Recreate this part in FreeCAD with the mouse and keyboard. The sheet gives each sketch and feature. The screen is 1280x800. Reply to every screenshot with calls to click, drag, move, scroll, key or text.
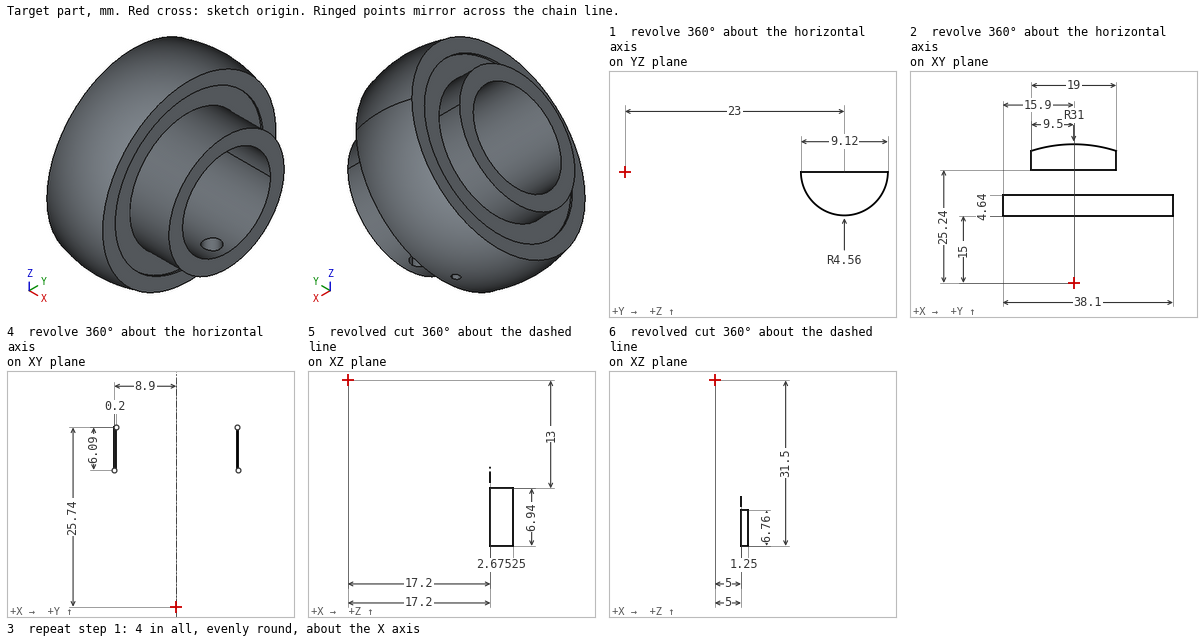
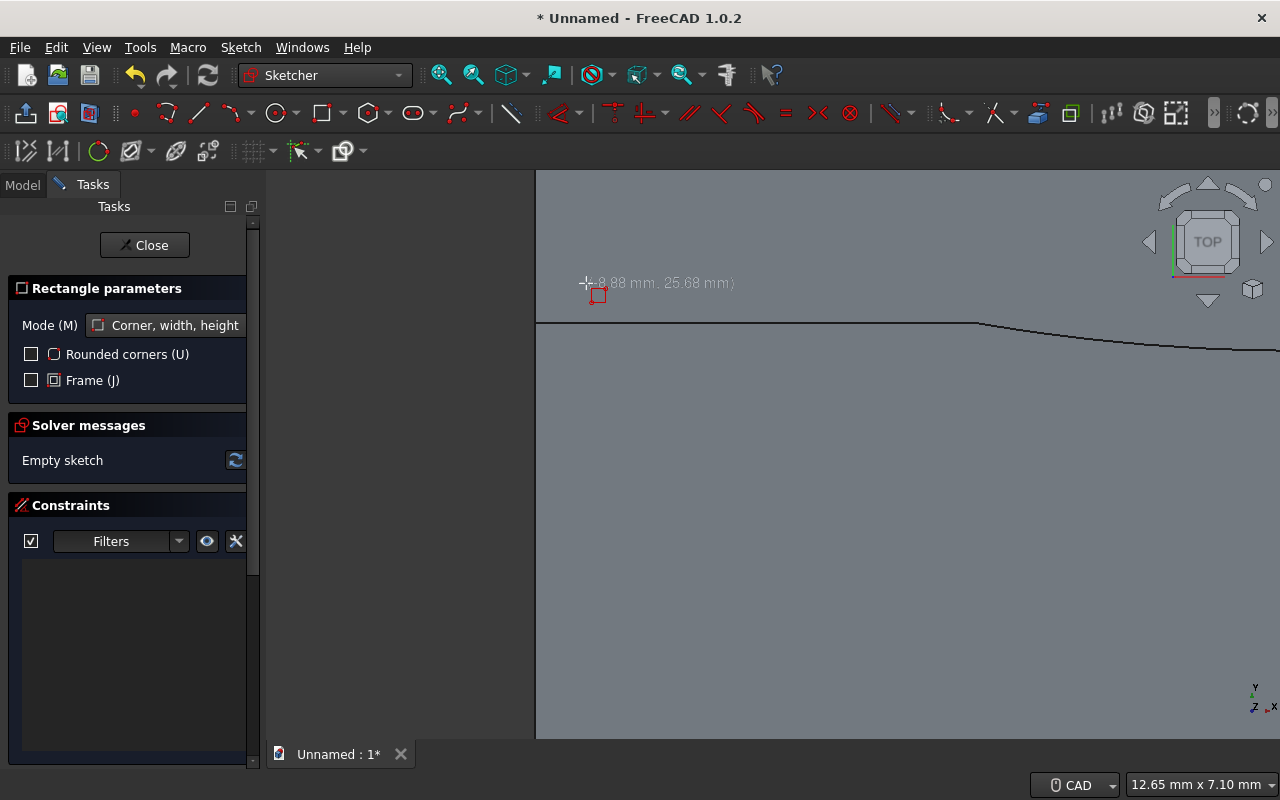
scroll(587, 284, down, 9)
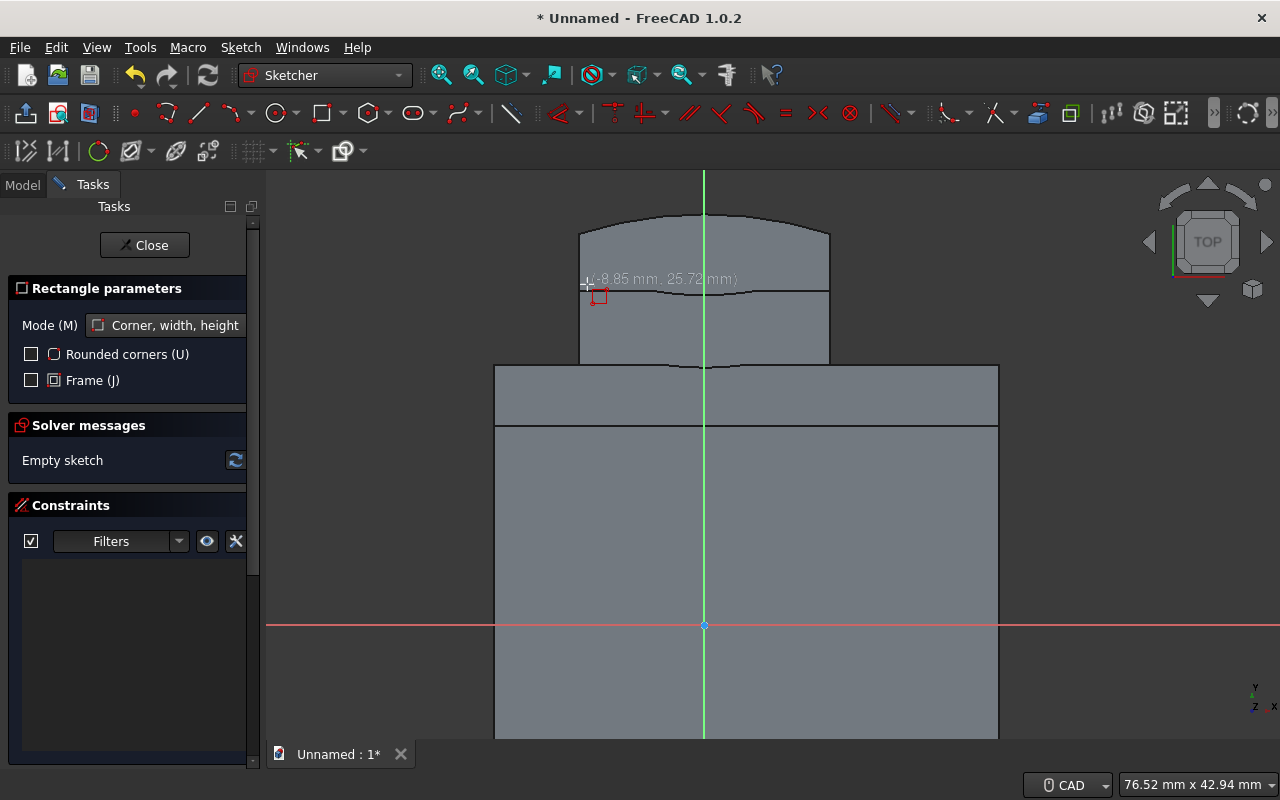
click(587, 284)
click(589, 365)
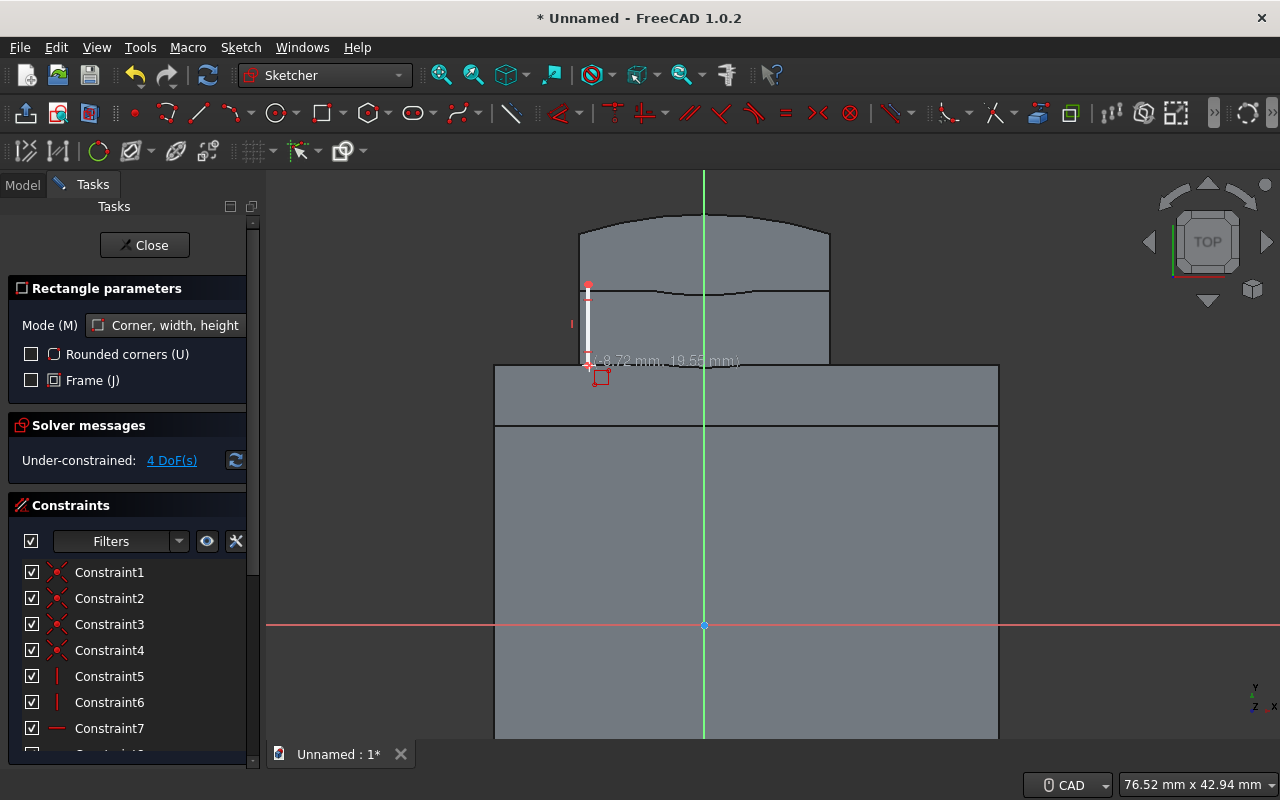
scroll(820, 284, up, 9)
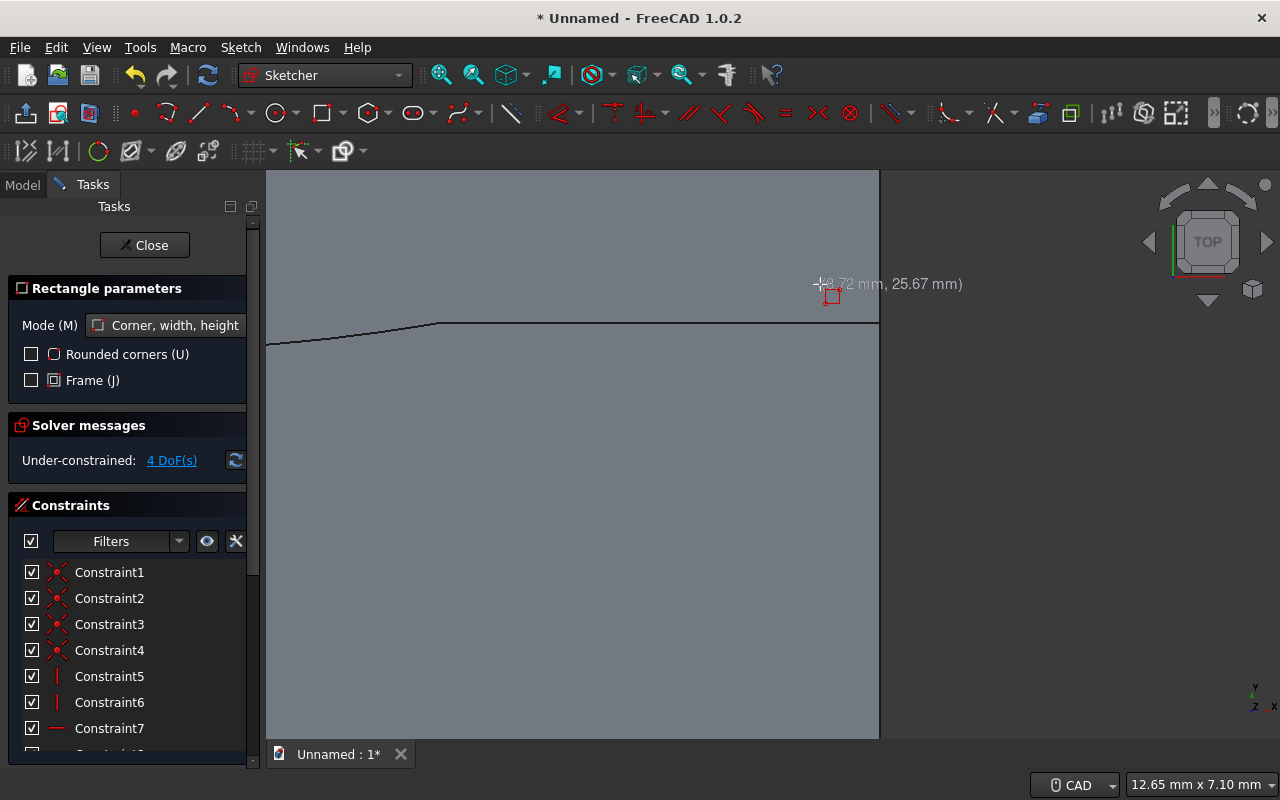
scroll(821, 284, down, 9)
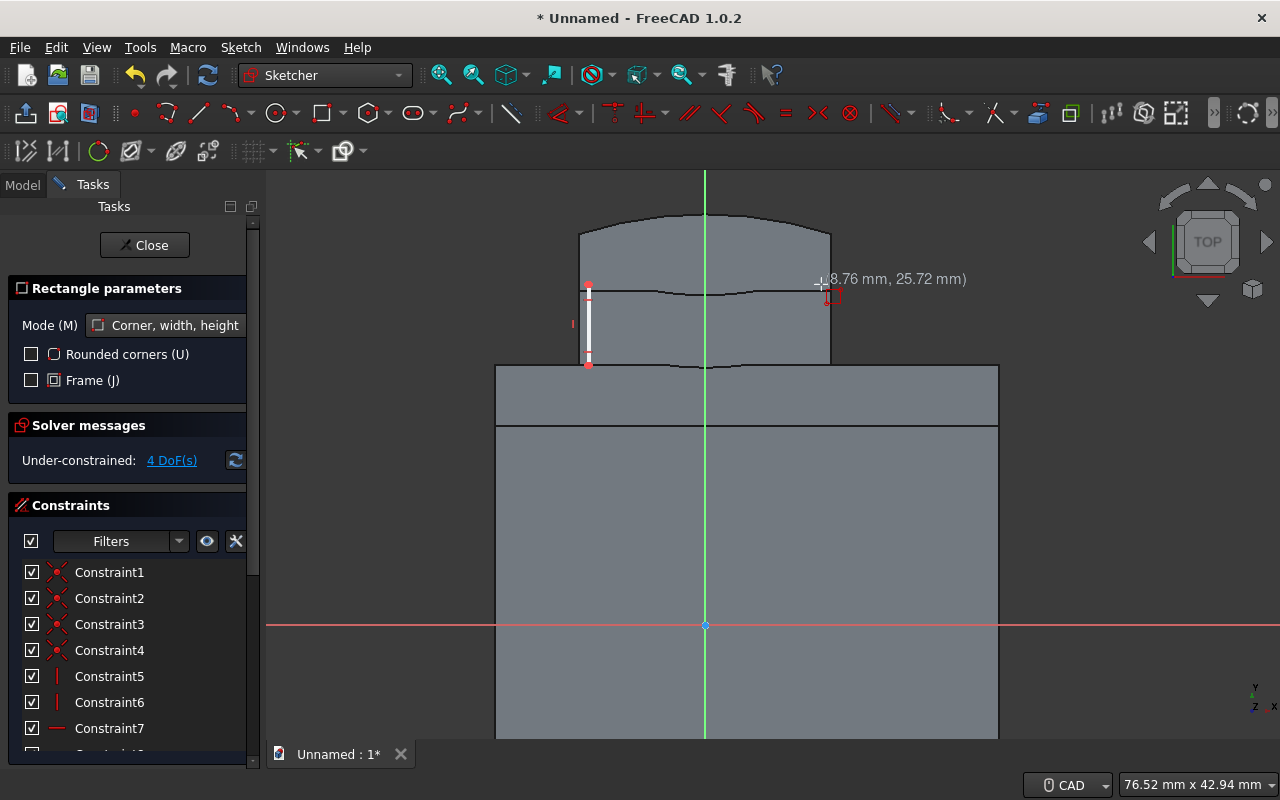
click(821, 284)
click(823, 365)
key(Escape)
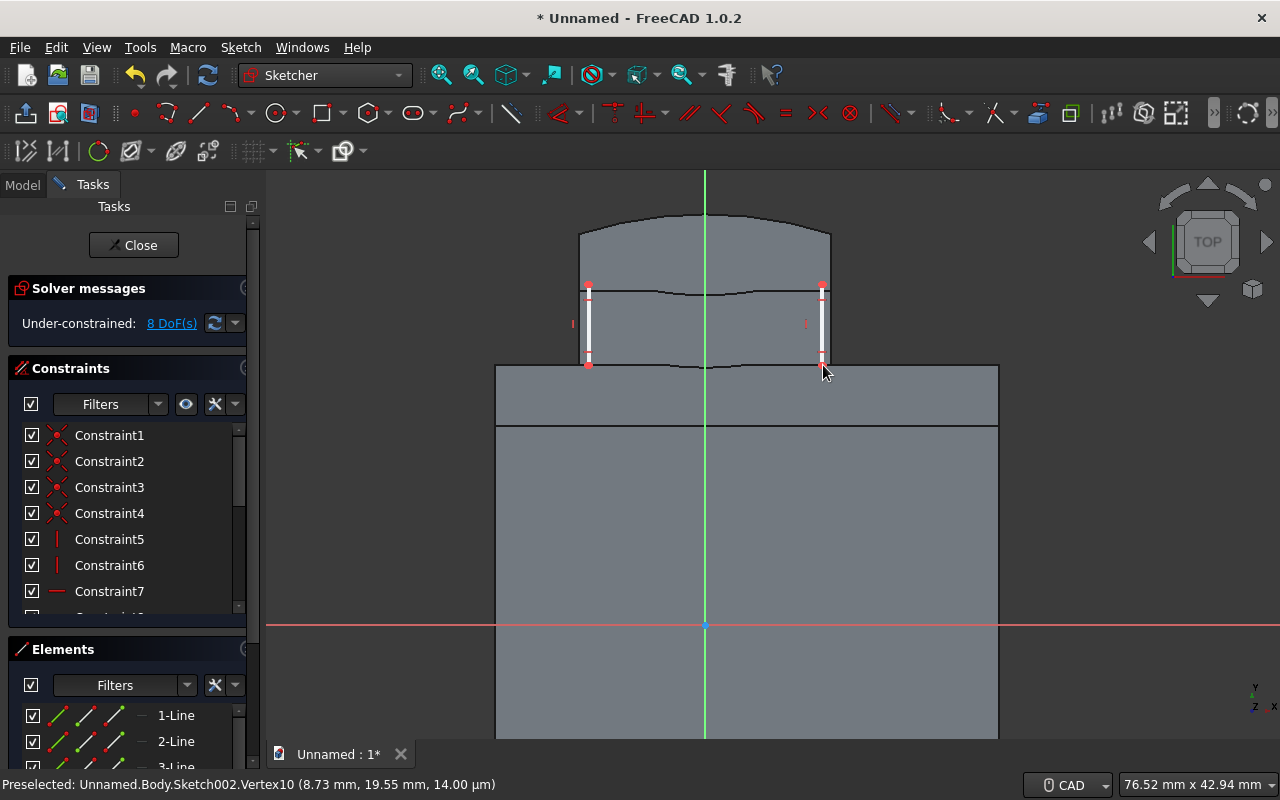
scroll(590, 285, up, 10)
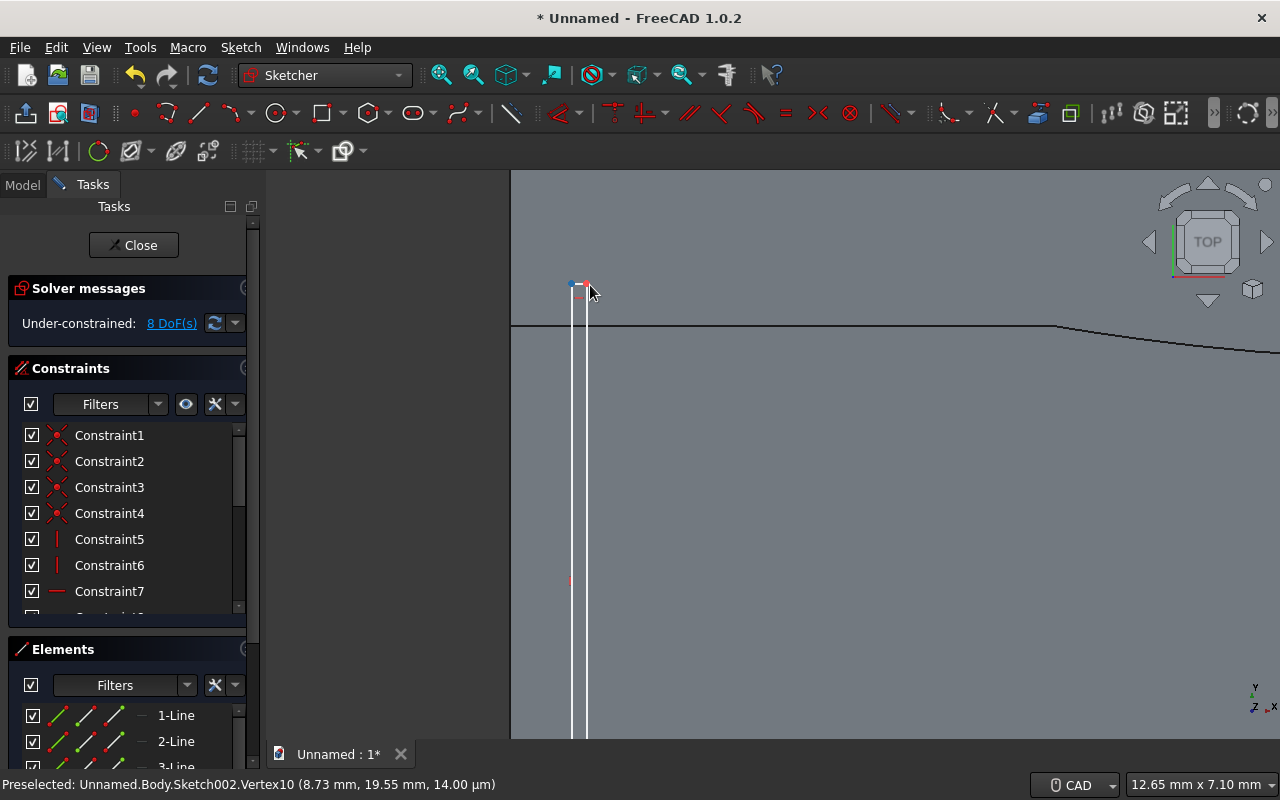
click(587, 284)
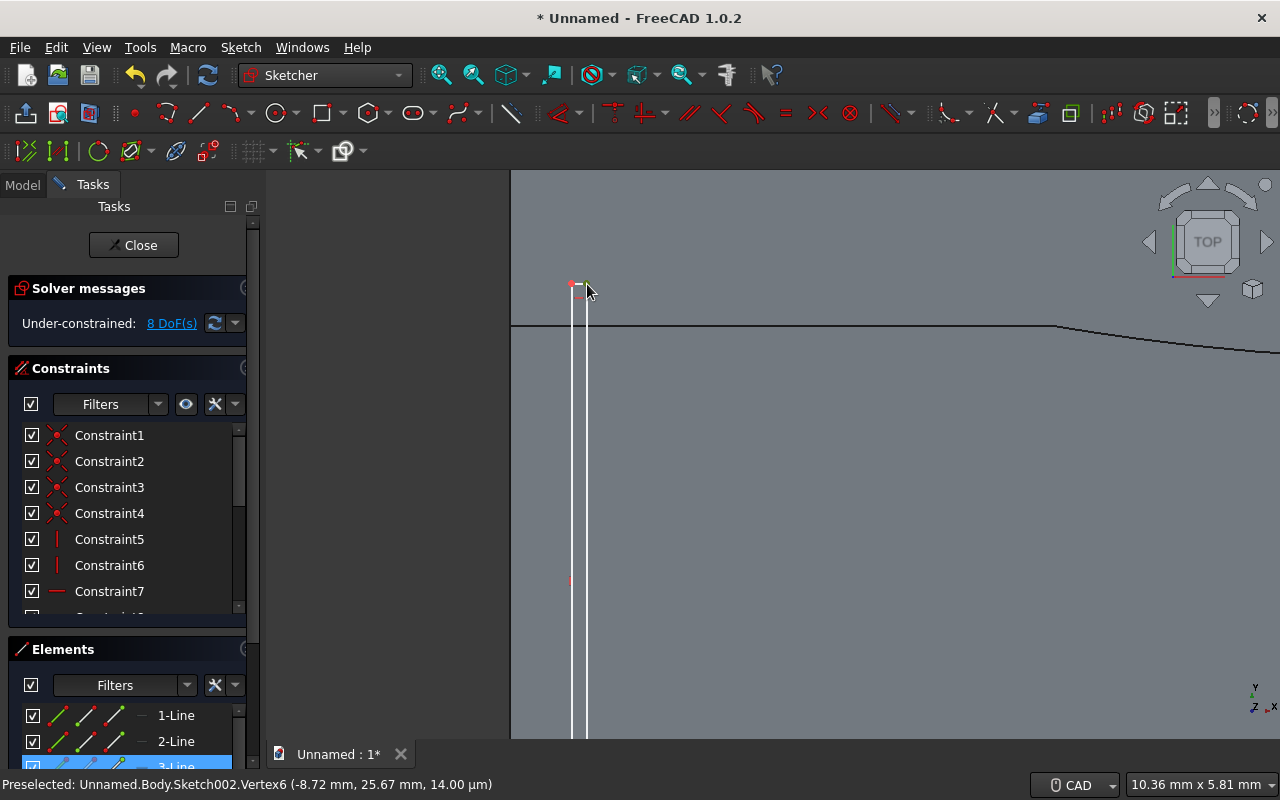
scroll(589, 285, down, 10)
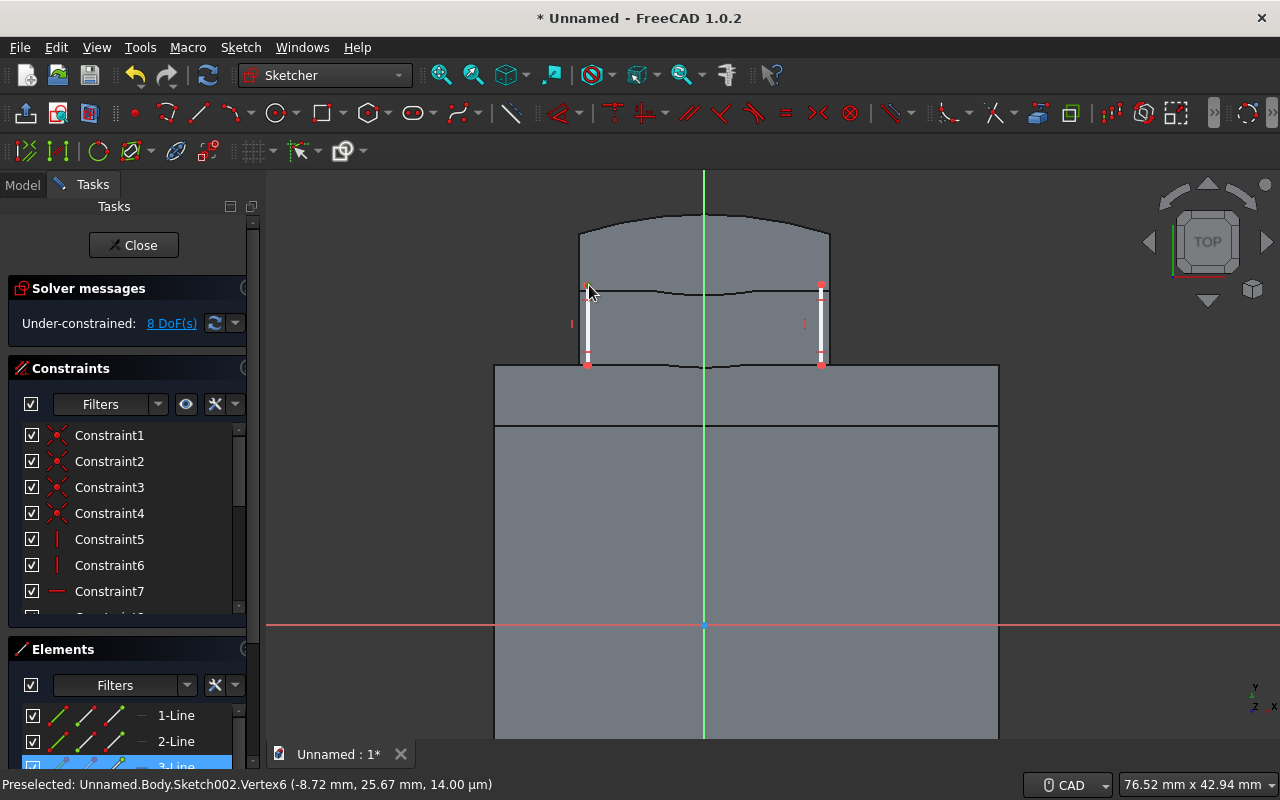
scroll(820, 285, up, 10)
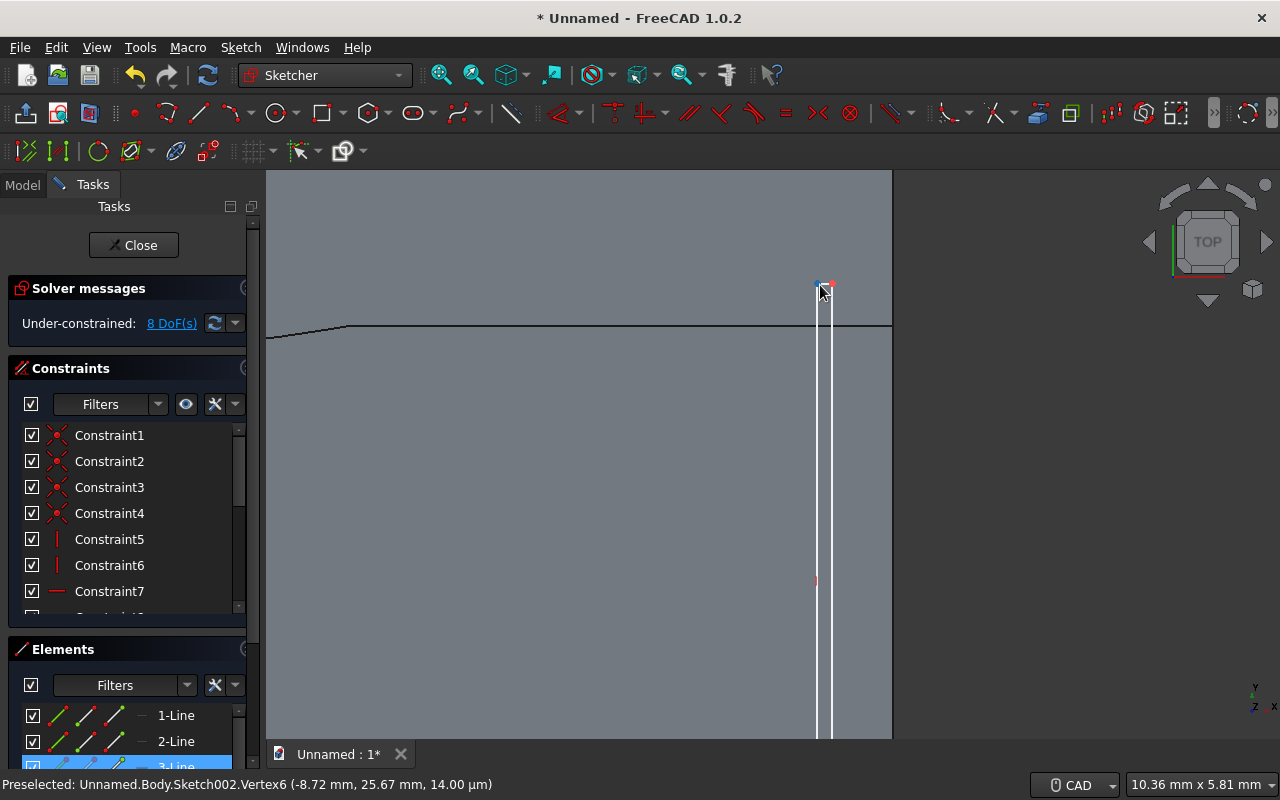
click(817, 284)